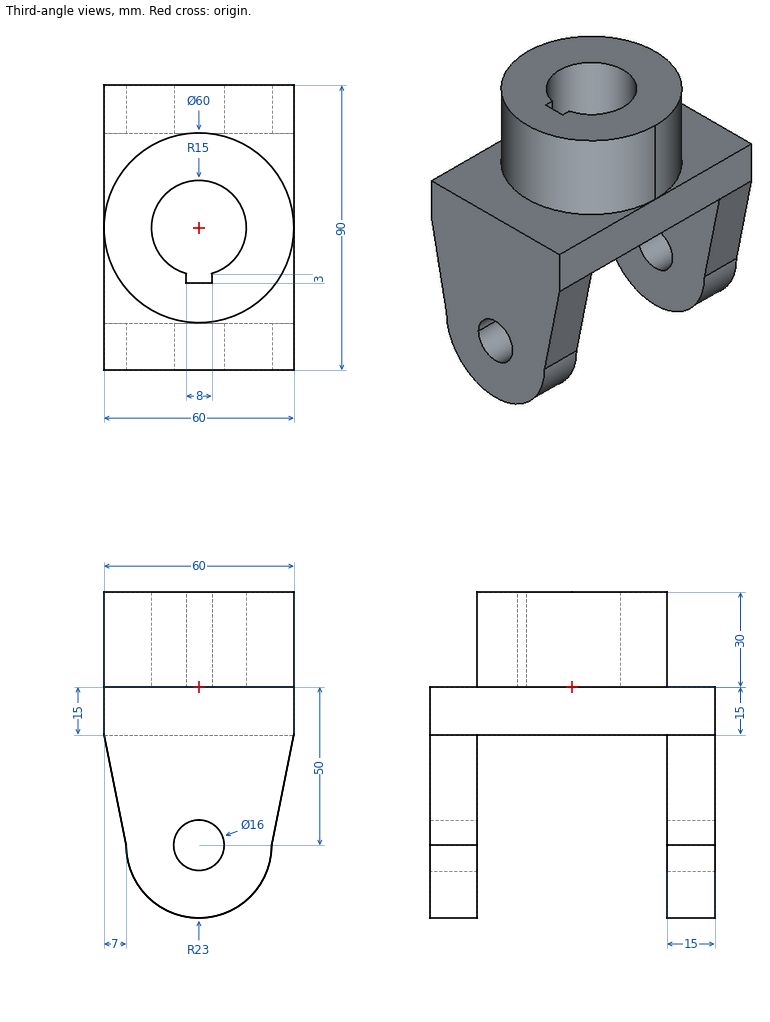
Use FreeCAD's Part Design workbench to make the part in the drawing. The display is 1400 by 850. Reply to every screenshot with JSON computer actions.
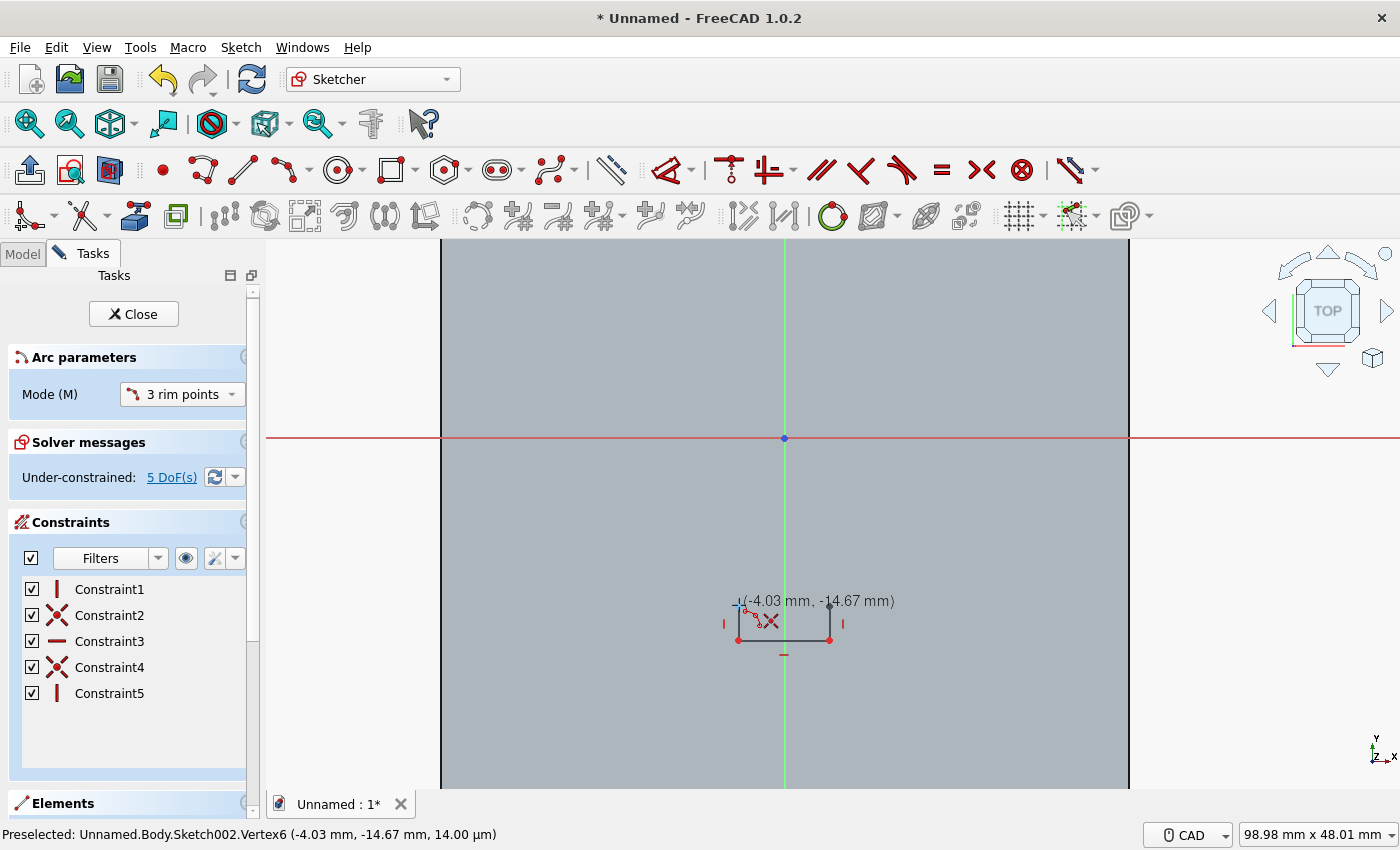
{"action": "left_click", "coordinate": [739, 606]}
{"action": "left_click", "coordinate": [830, 606]}
{"action": "left_click", "coordinate": [878, 294]}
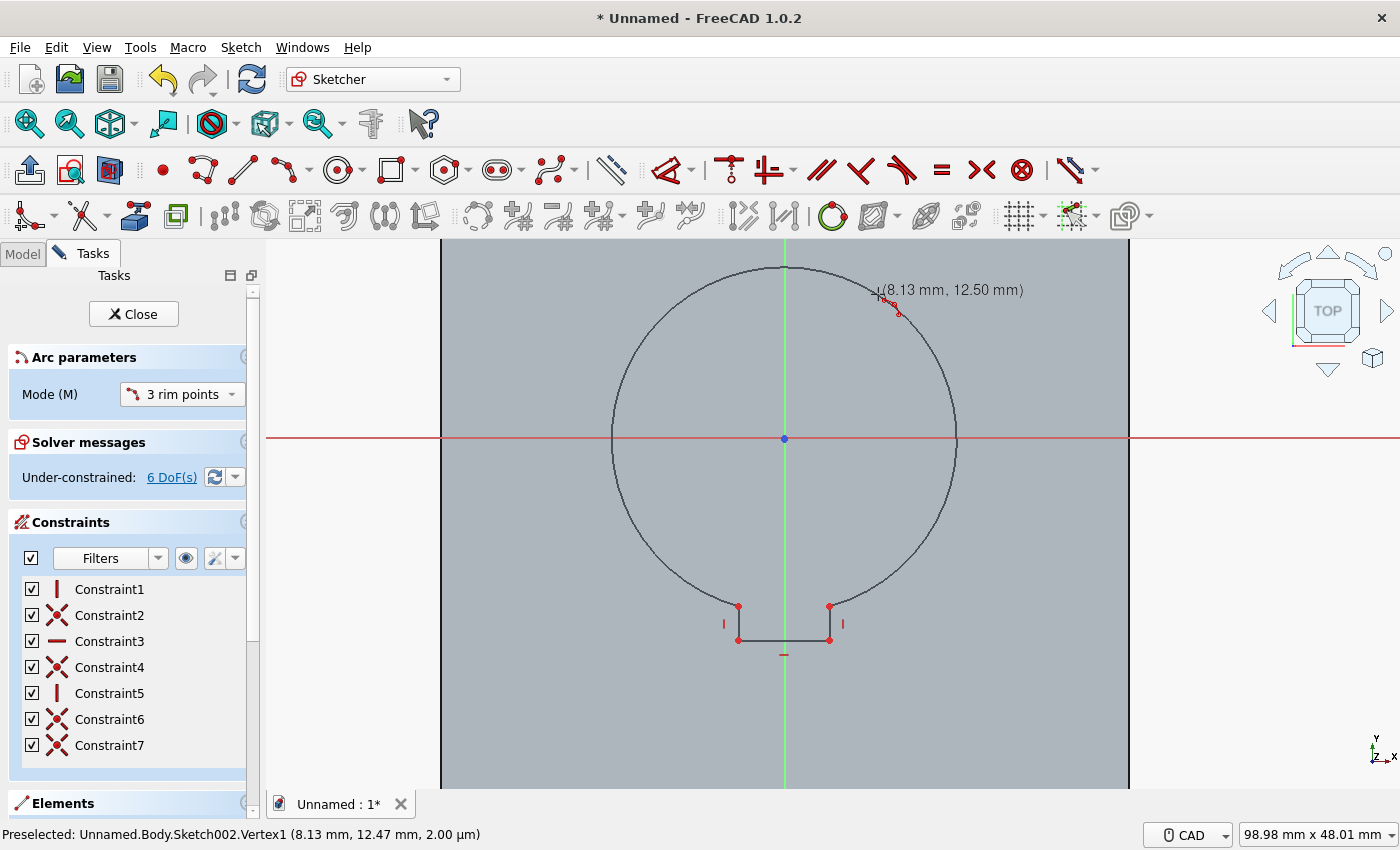
{"action": "left_click", "coordinate": [338, 170]}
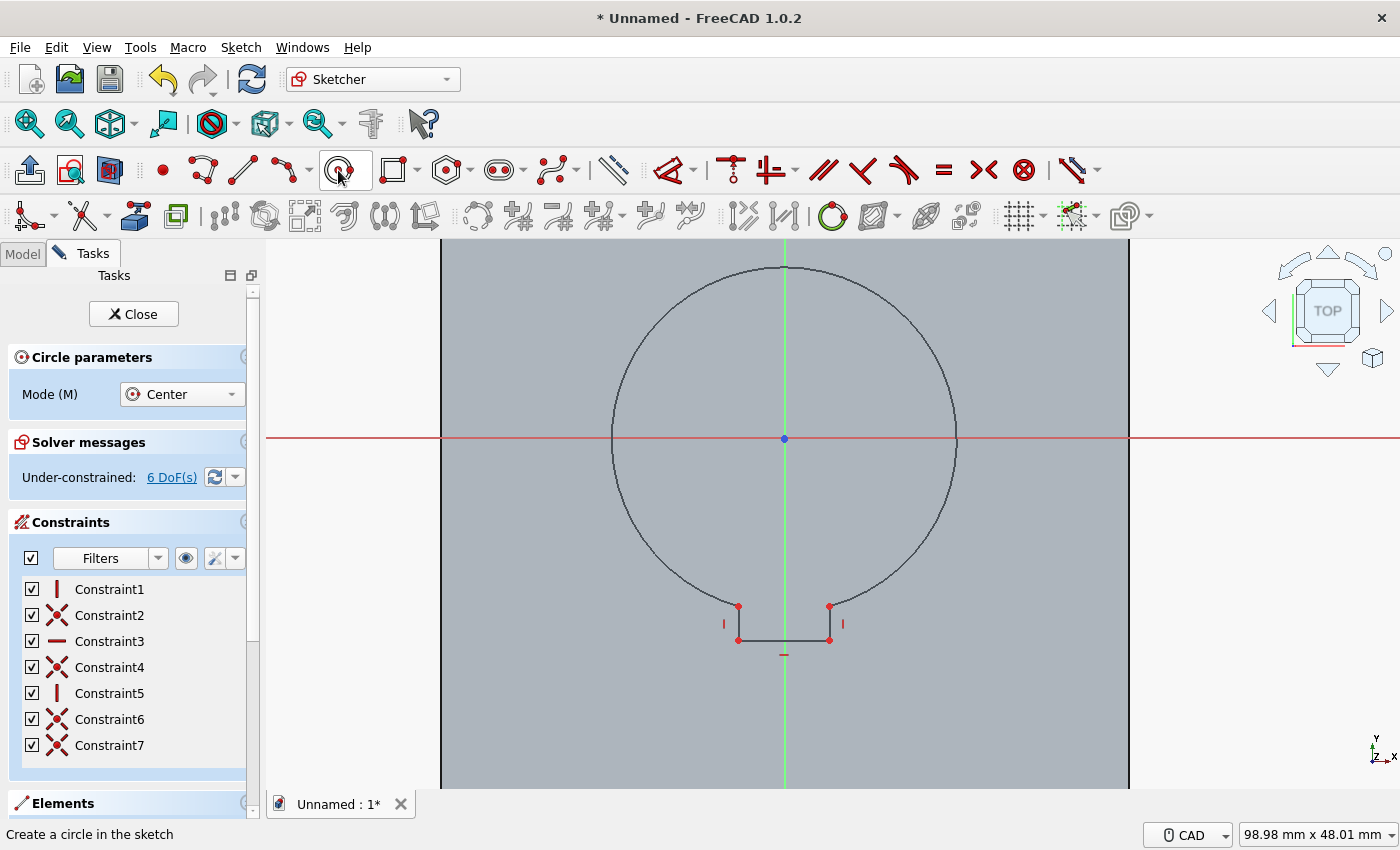
{"action": "left_click", "coordinate": [785, 438]}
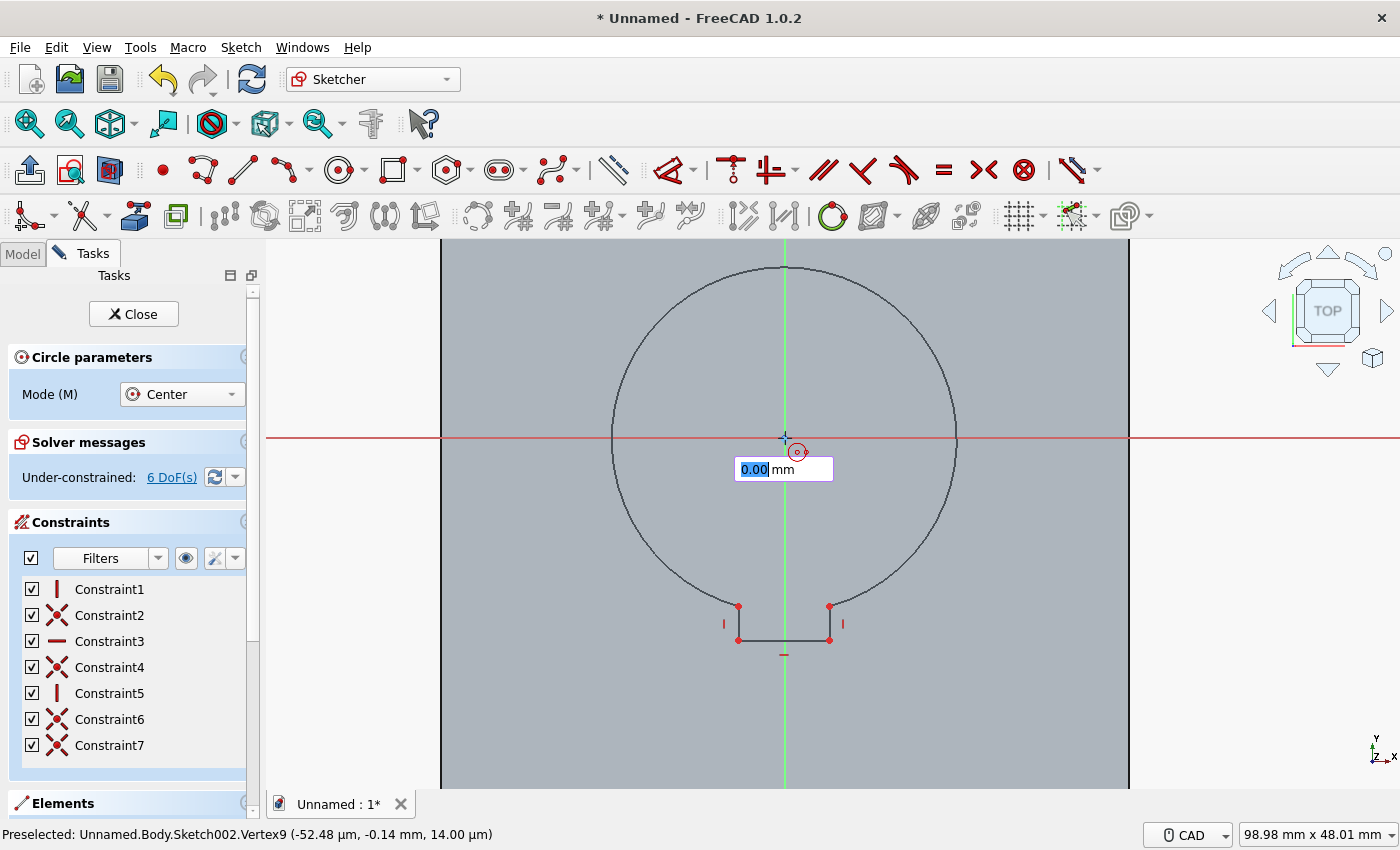
{"action": "scroll", "coordinate": [740, 606], "scroll_direction": "down", "scroll_amount": 3}
{"action": "mouse_move", "coordinate": [898, 381]}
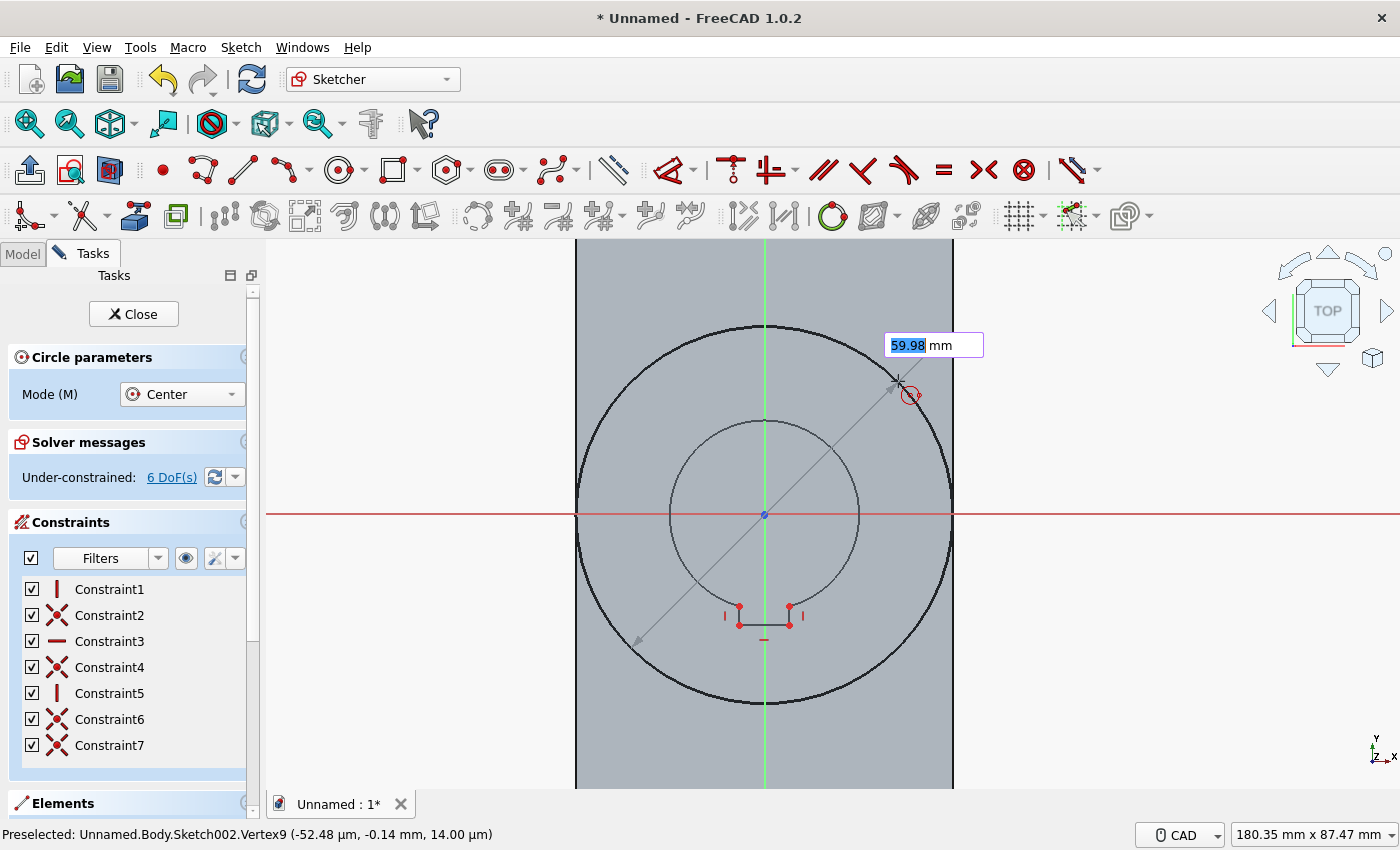
{"action": "type", "text": "60"}
{"action": "key", "text": "Return"}
{"action": "key", "text": "Escape"}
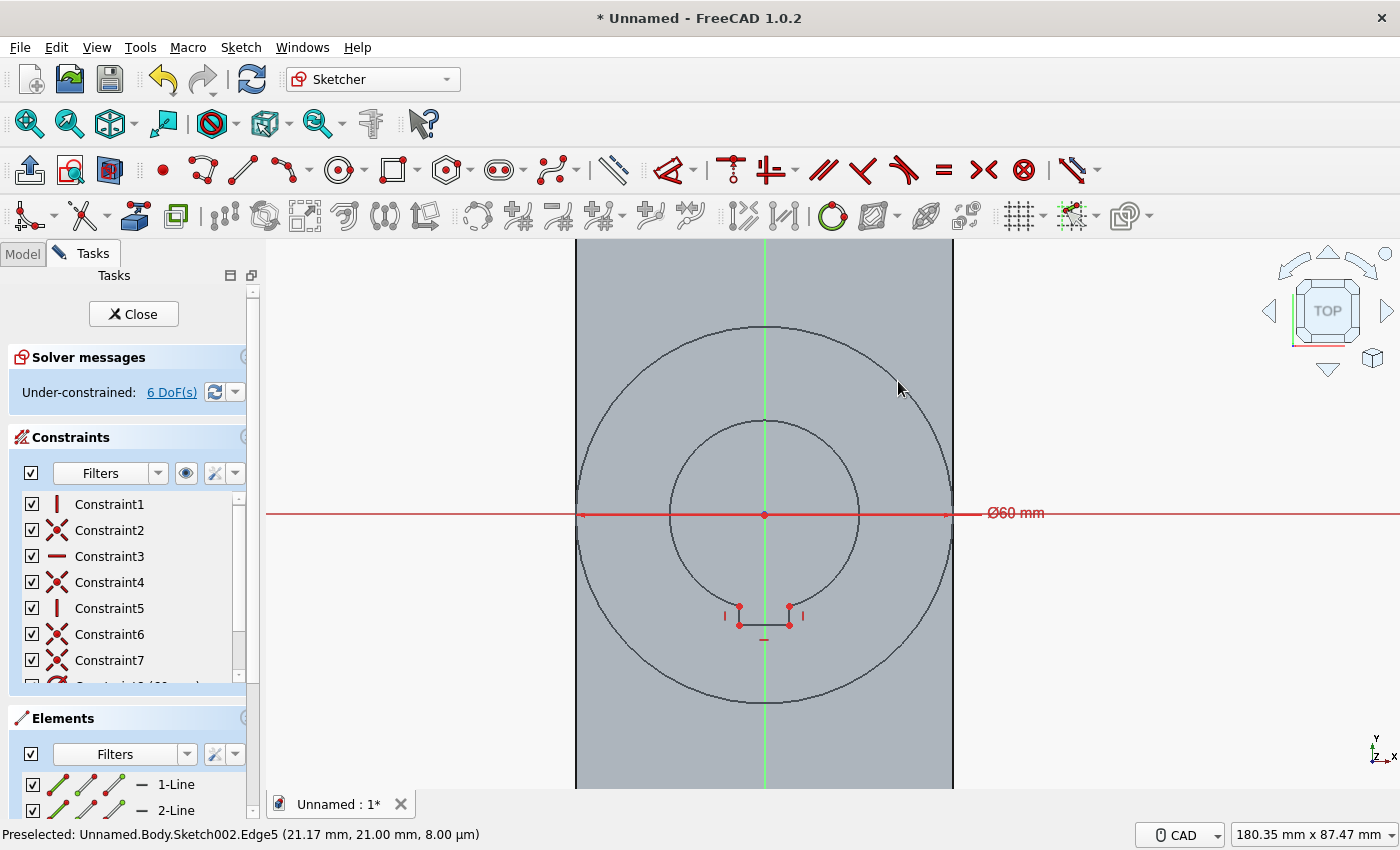
{"action": "left_click_drag", "start_coordinate": [754, 504], "coordinate": [775, 525]}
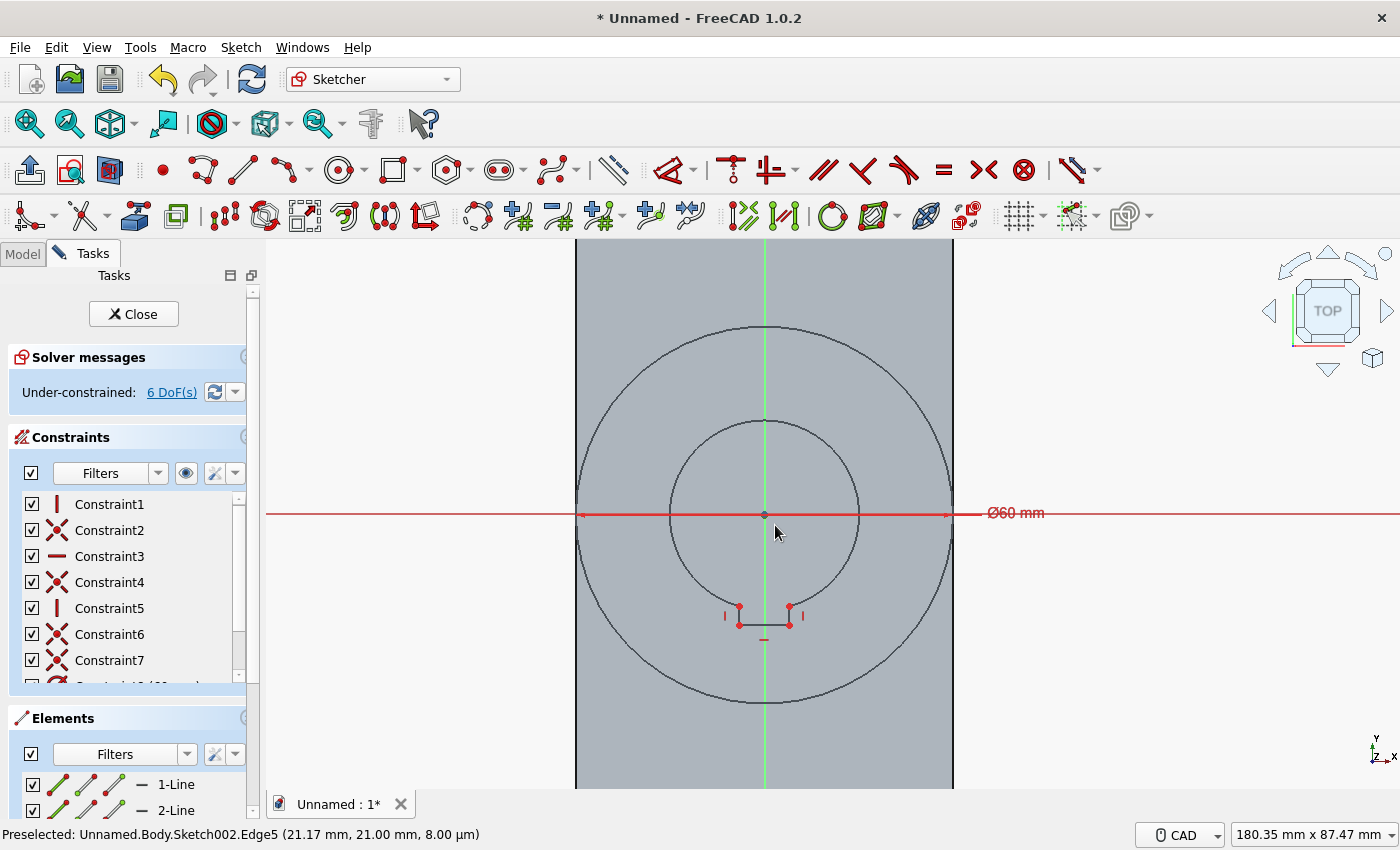
{"action": "left_click", "coordinate": [732, 170]}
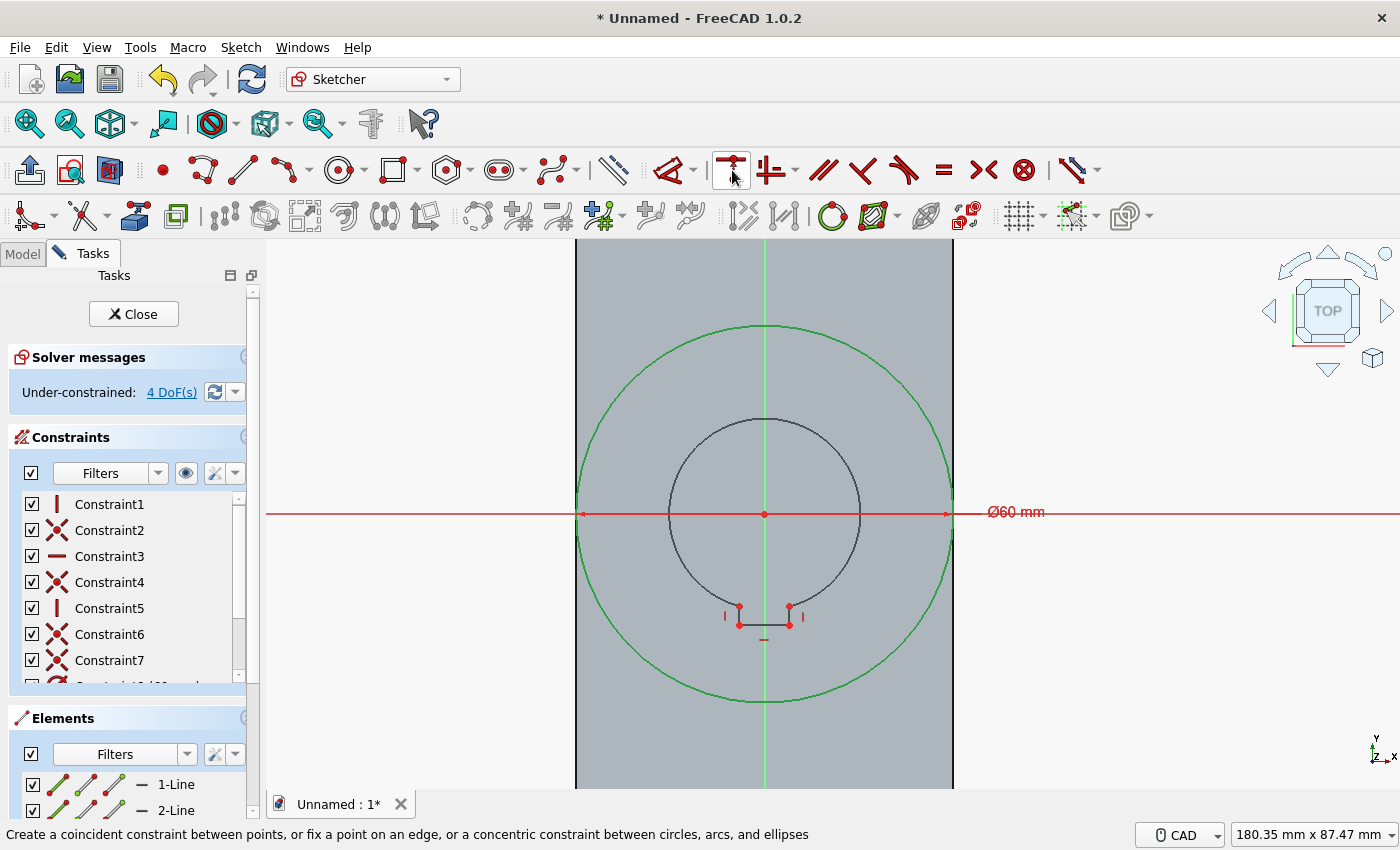
{"action": "left_click", "coordinate": [668, 170]}